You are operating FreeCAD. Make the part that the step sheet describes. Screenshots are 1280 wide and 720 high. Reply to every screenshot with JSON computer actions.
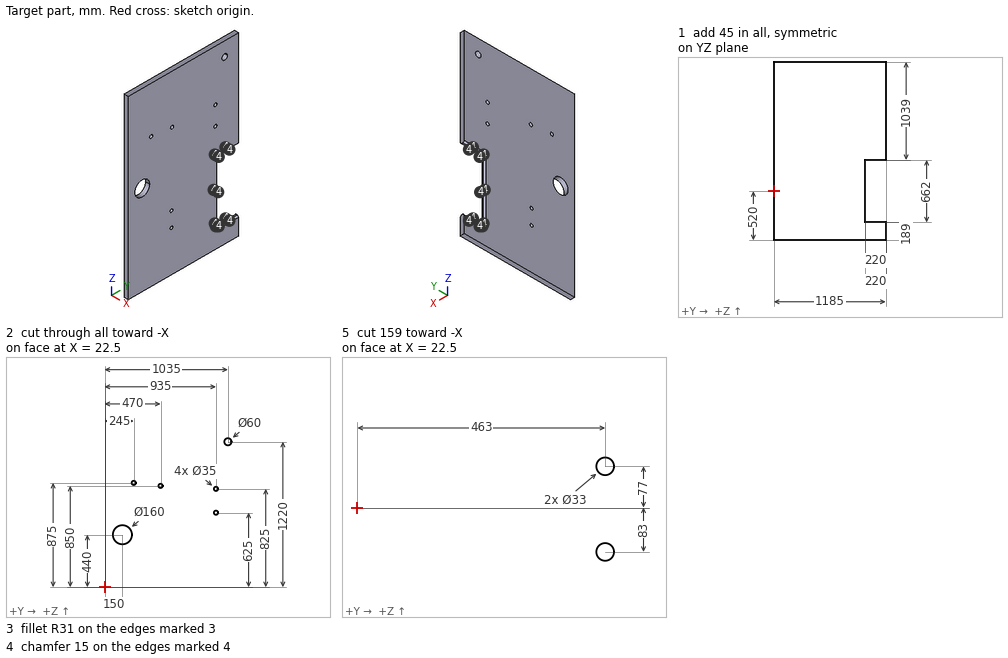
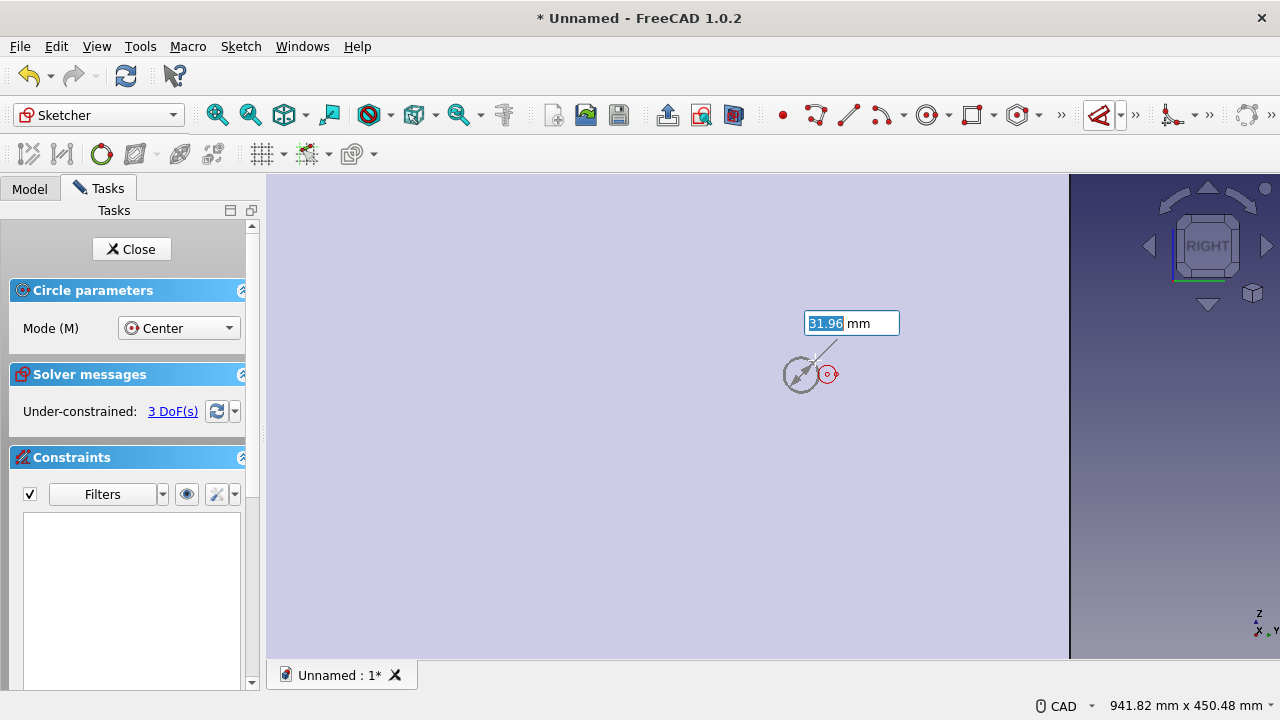
{"action": "left_click", "coordinate": [815, 359]}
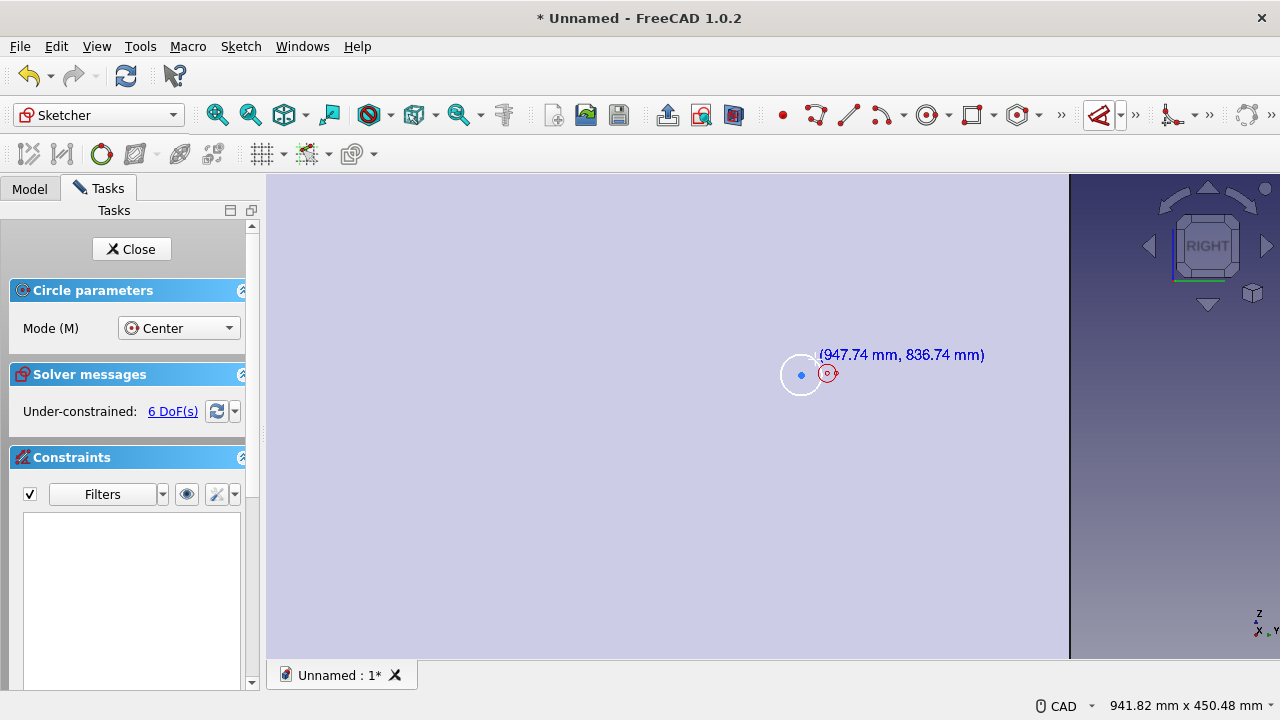
{"action": "scroll", "coordinate": [815, 360], "scroll_direction": "down", "scroll_amount": 7}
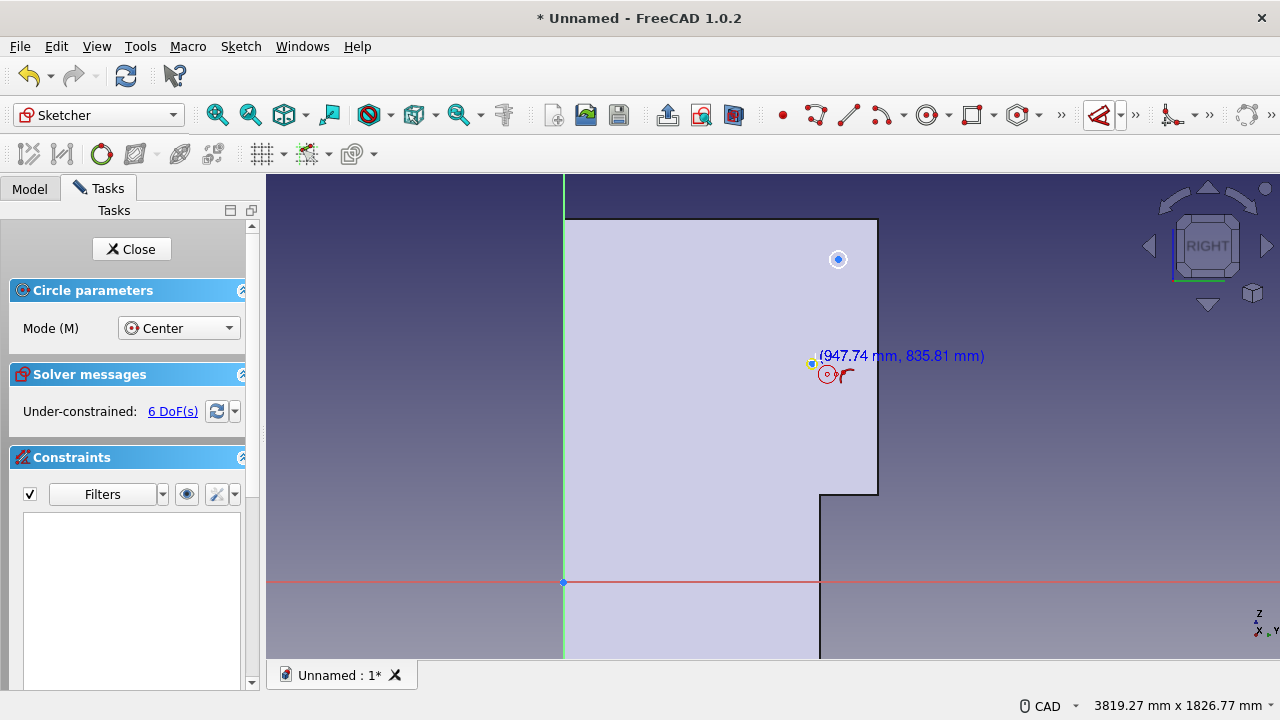
{"action": "left_click", "coordinate": [812, 417]}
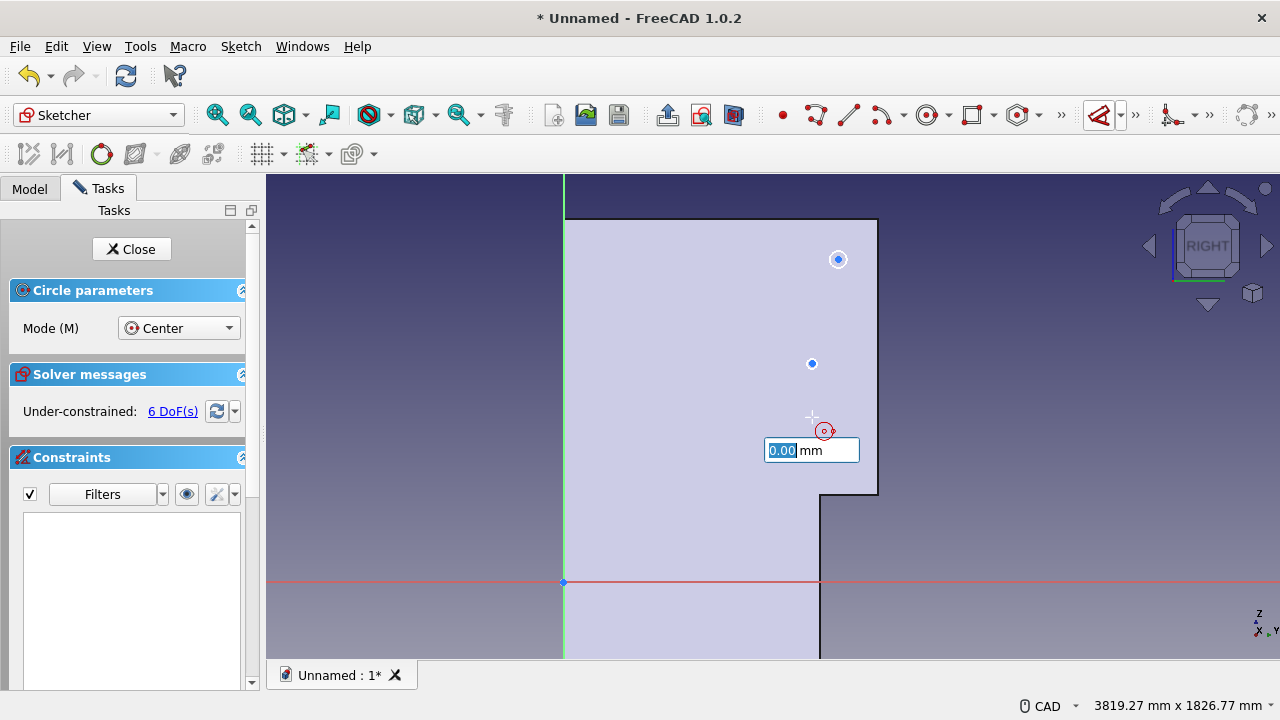
{"action": "scroll", "coordinate": [815, 413], "scroll_direction": "up", "scroll_amount": 7}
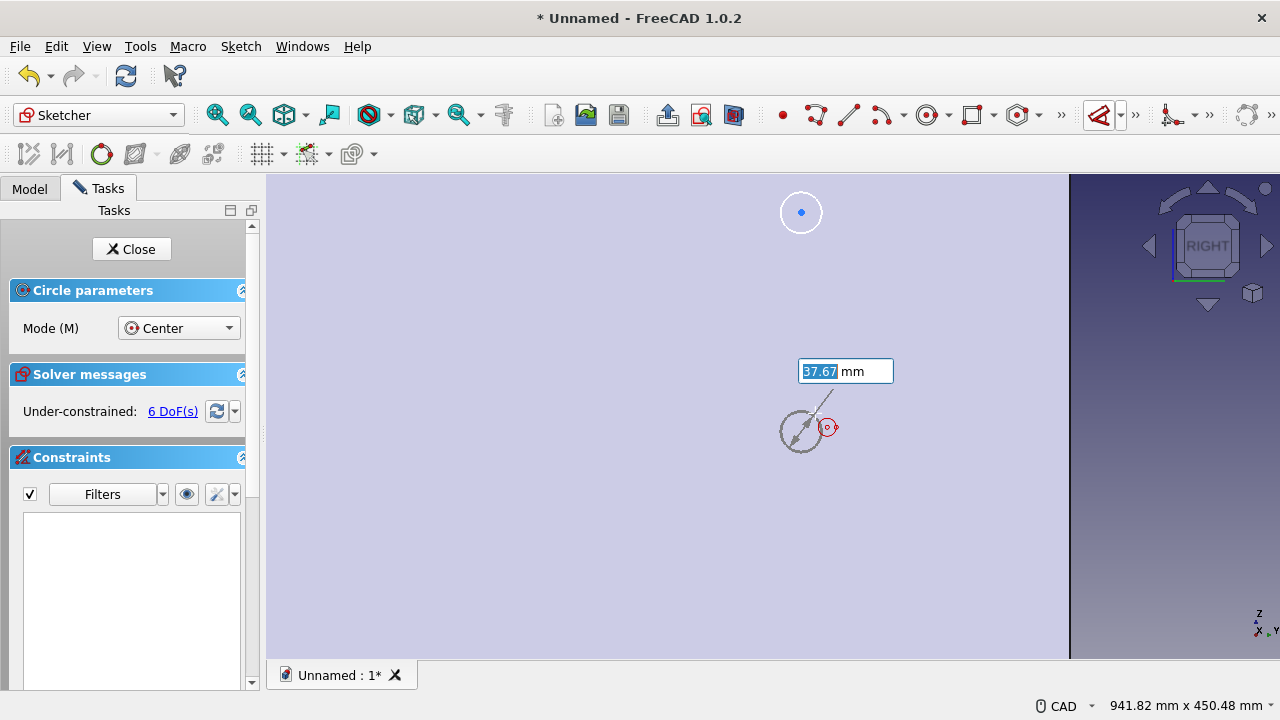
{"action": "left_click", "coordinate": [815, 412]}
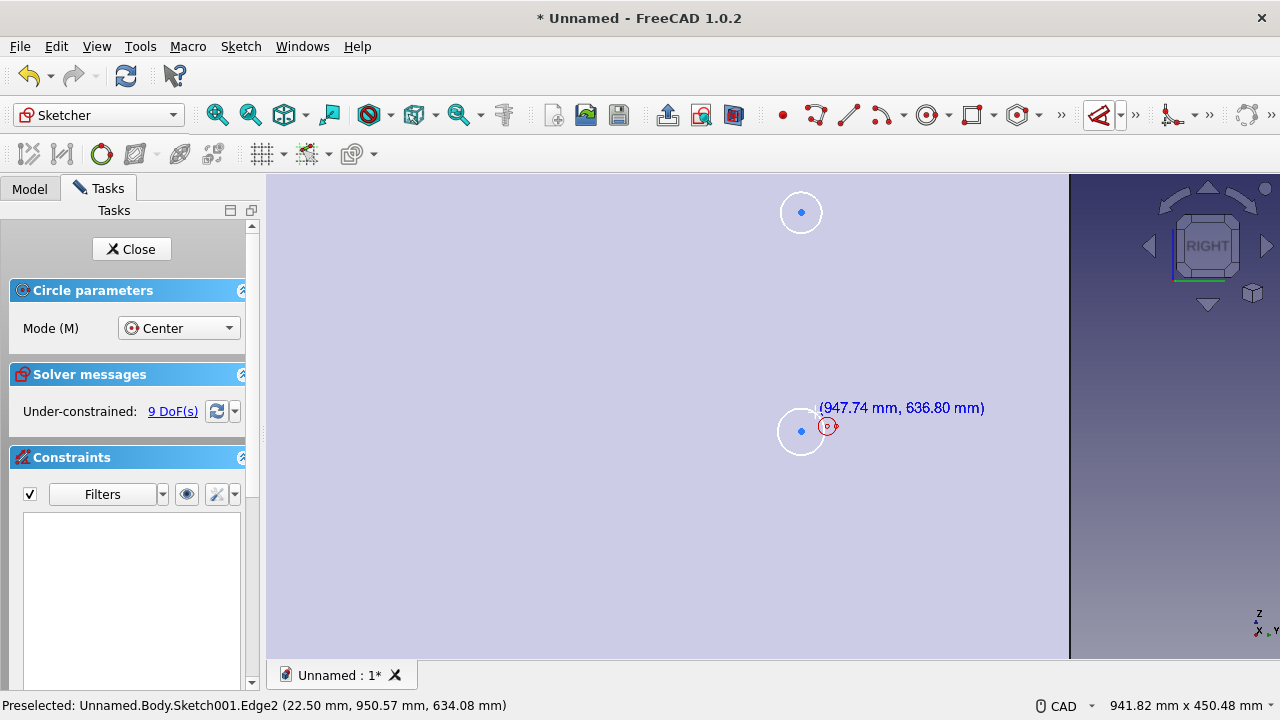
{"action": "scroll", "coordinate": [815, 413], "scroll_direction": "down", "scroll_amount": 7}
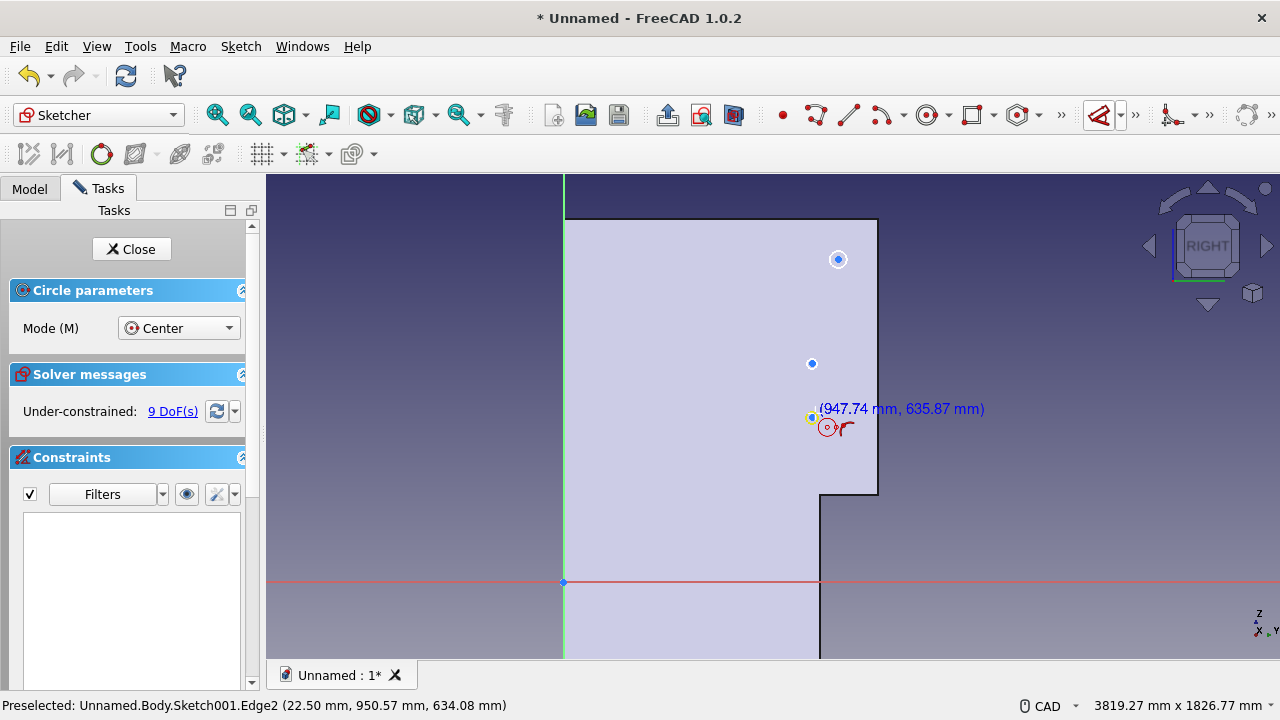
{"action": "scroll", "coordinate": [689, 357], "scroll_direction": "up", "scroll_amount": 8}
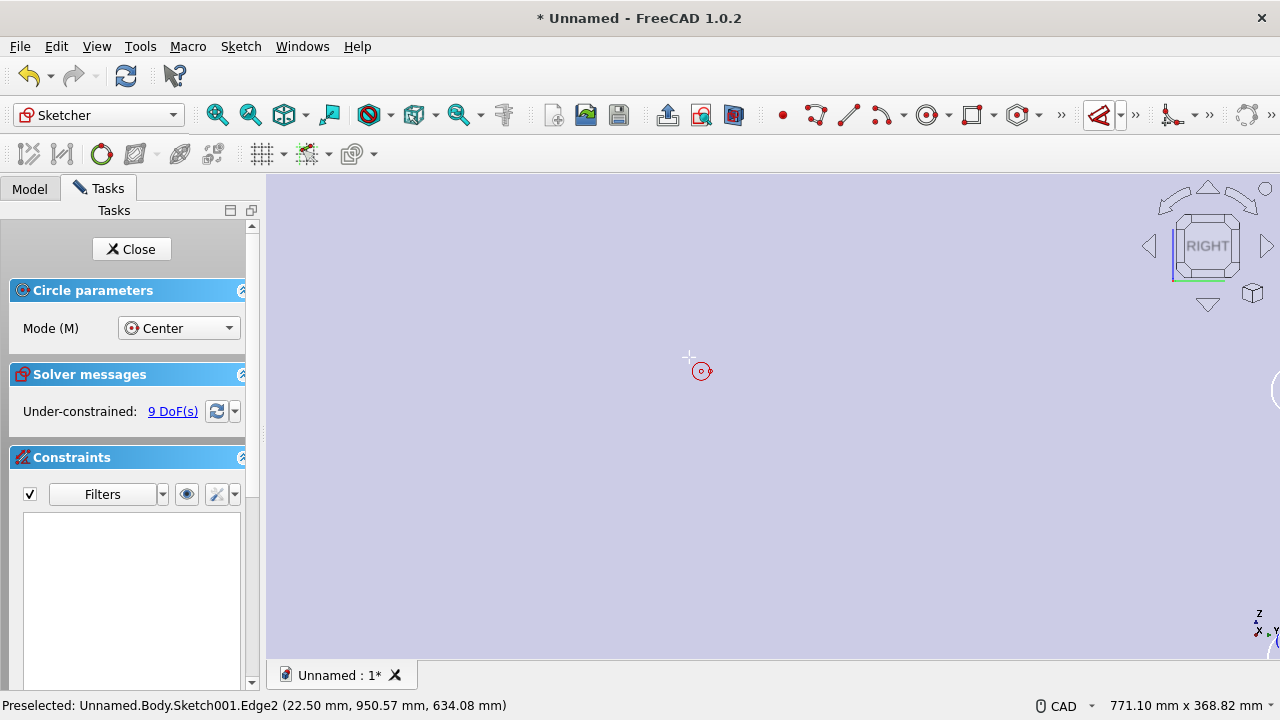
{"action": "scroll", "coordinate": [689, 357], "scroll_direction": "down", "scroll_amount": 8}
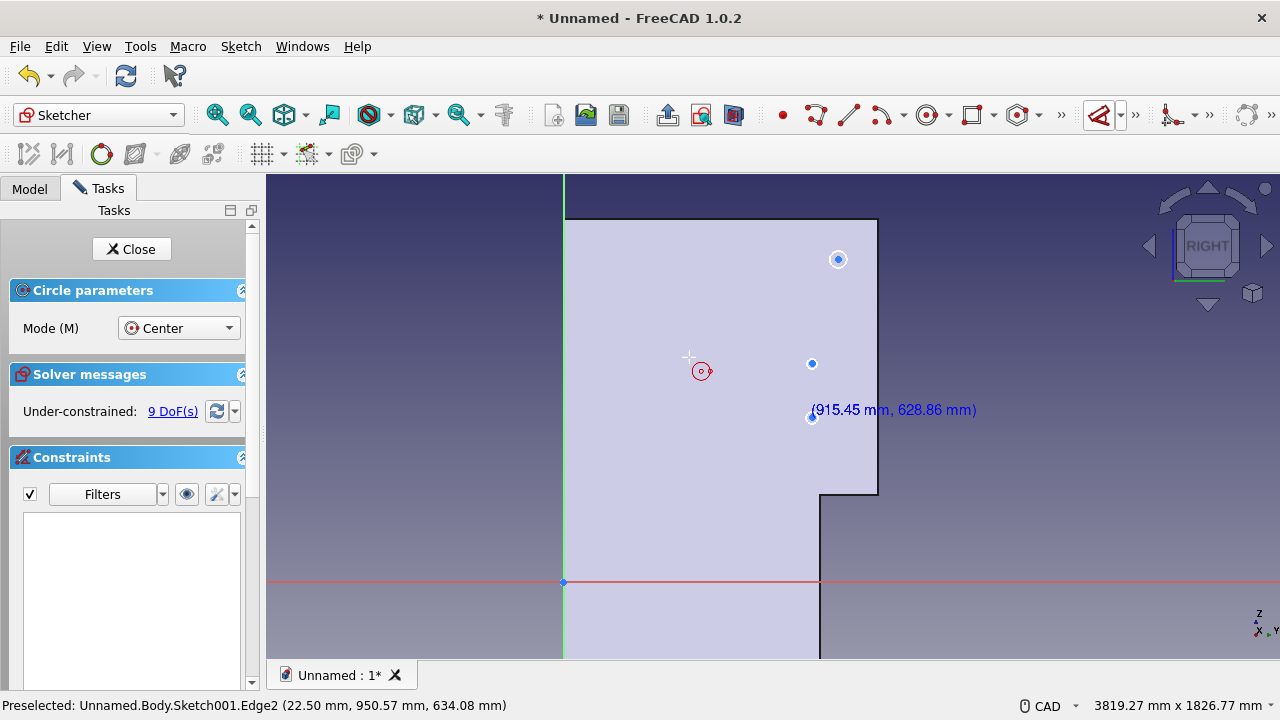
{"action": "left_click", "coordinate": [689, 357]}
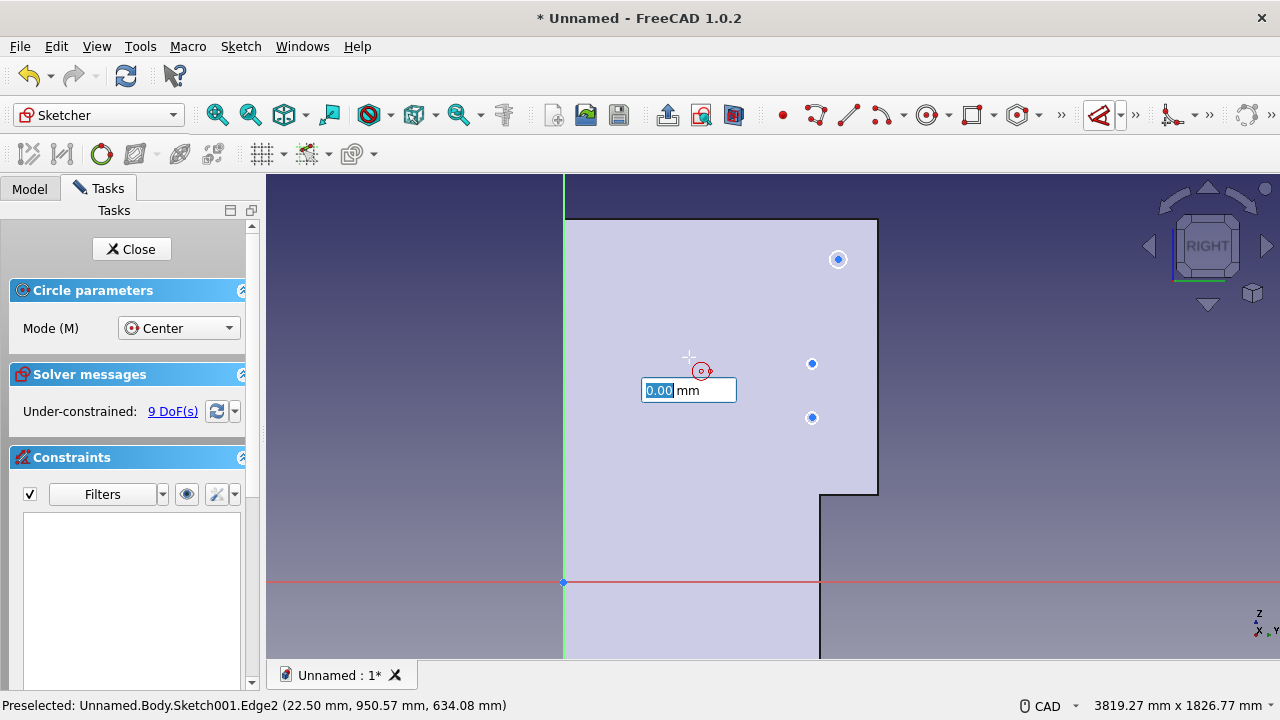
{"action": "scroll", "coordinate": [692, 353], "scroll_direction": "up", "scroll_amount": 7}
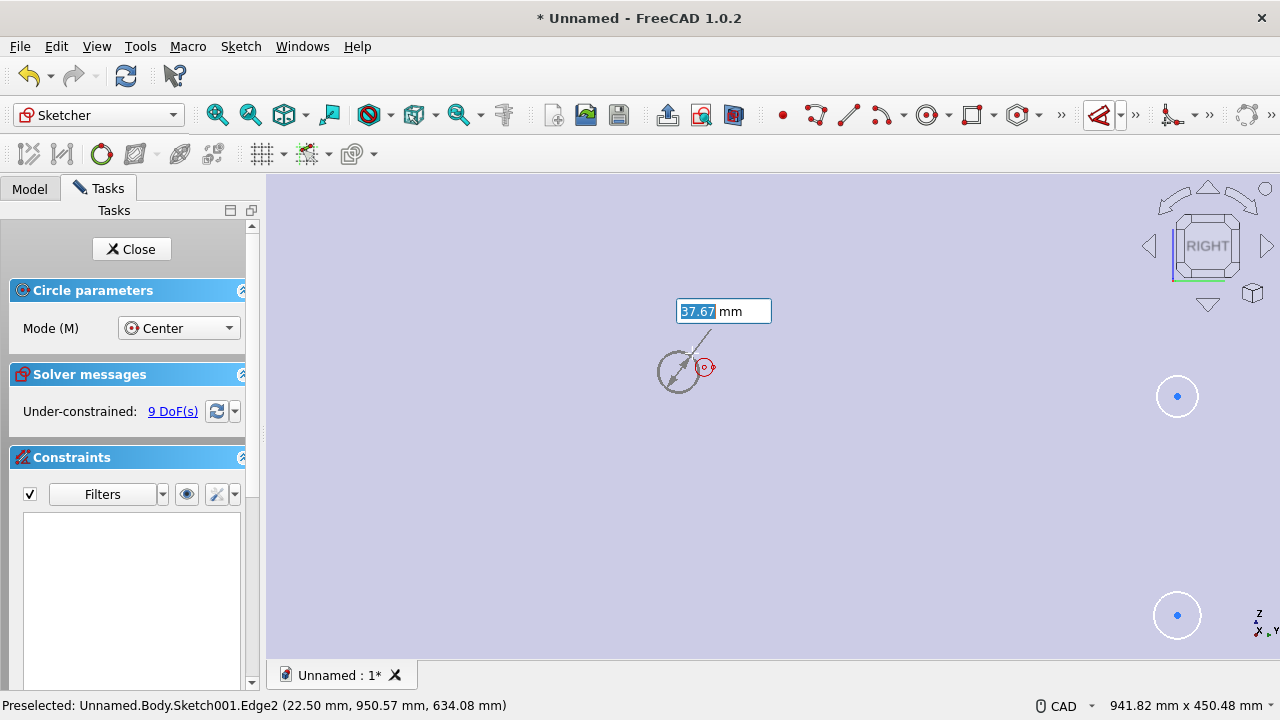
{"action": "left_click", "coordinate": [690, 354]}